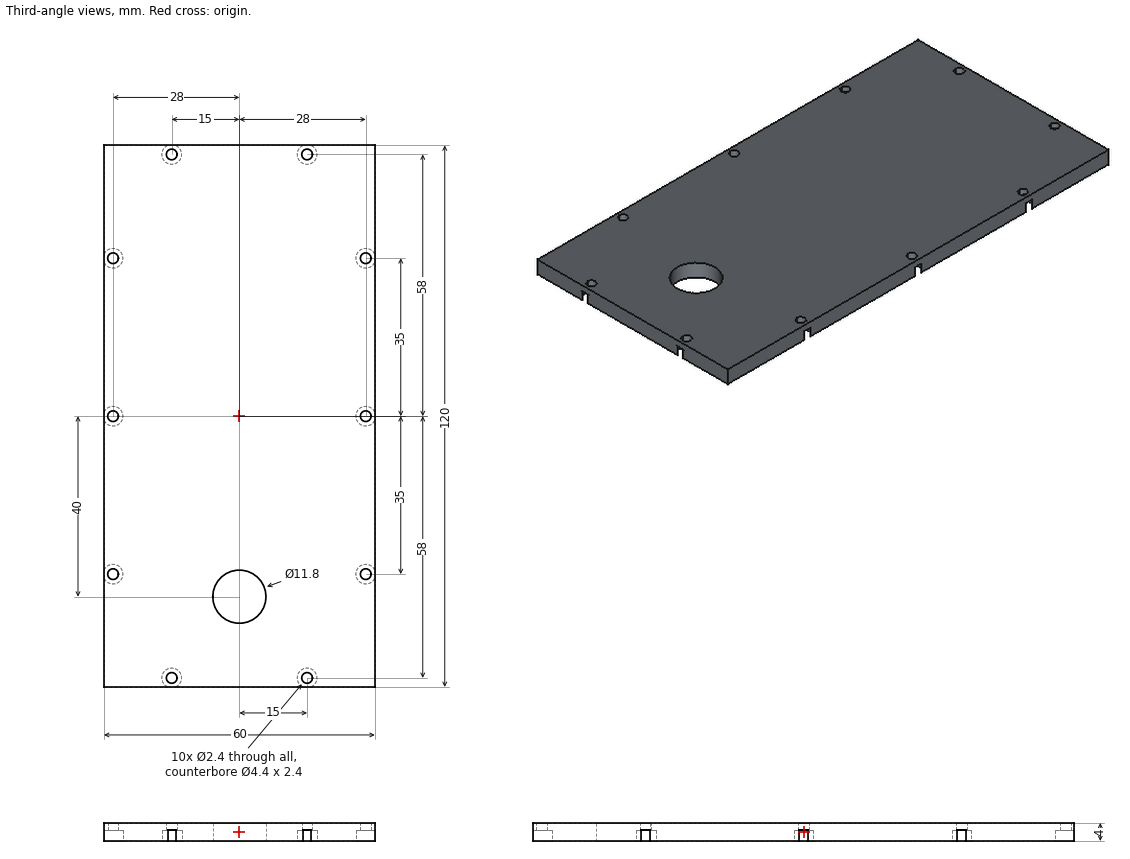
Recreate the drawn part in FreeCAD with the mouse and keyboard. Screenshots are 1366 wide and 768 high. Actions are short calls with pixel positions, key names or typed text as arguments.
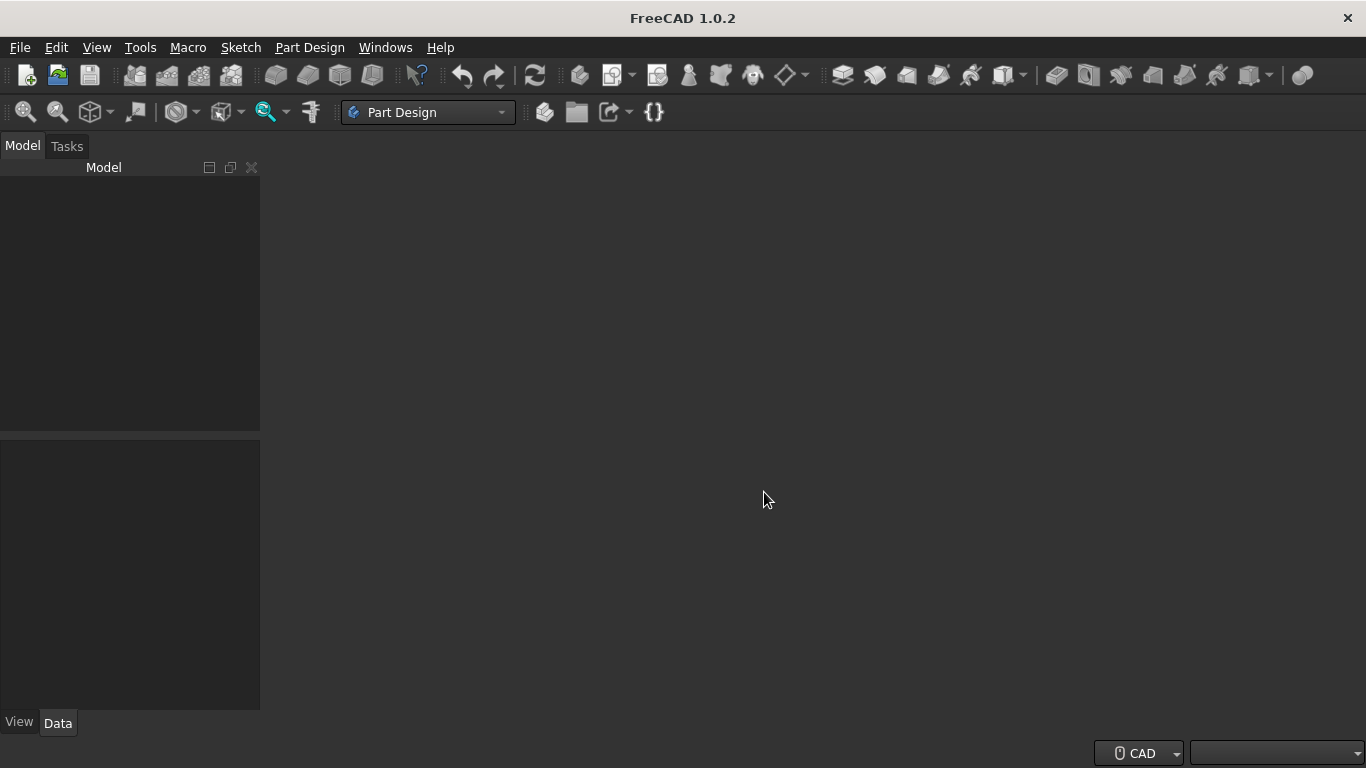
click(26, 76)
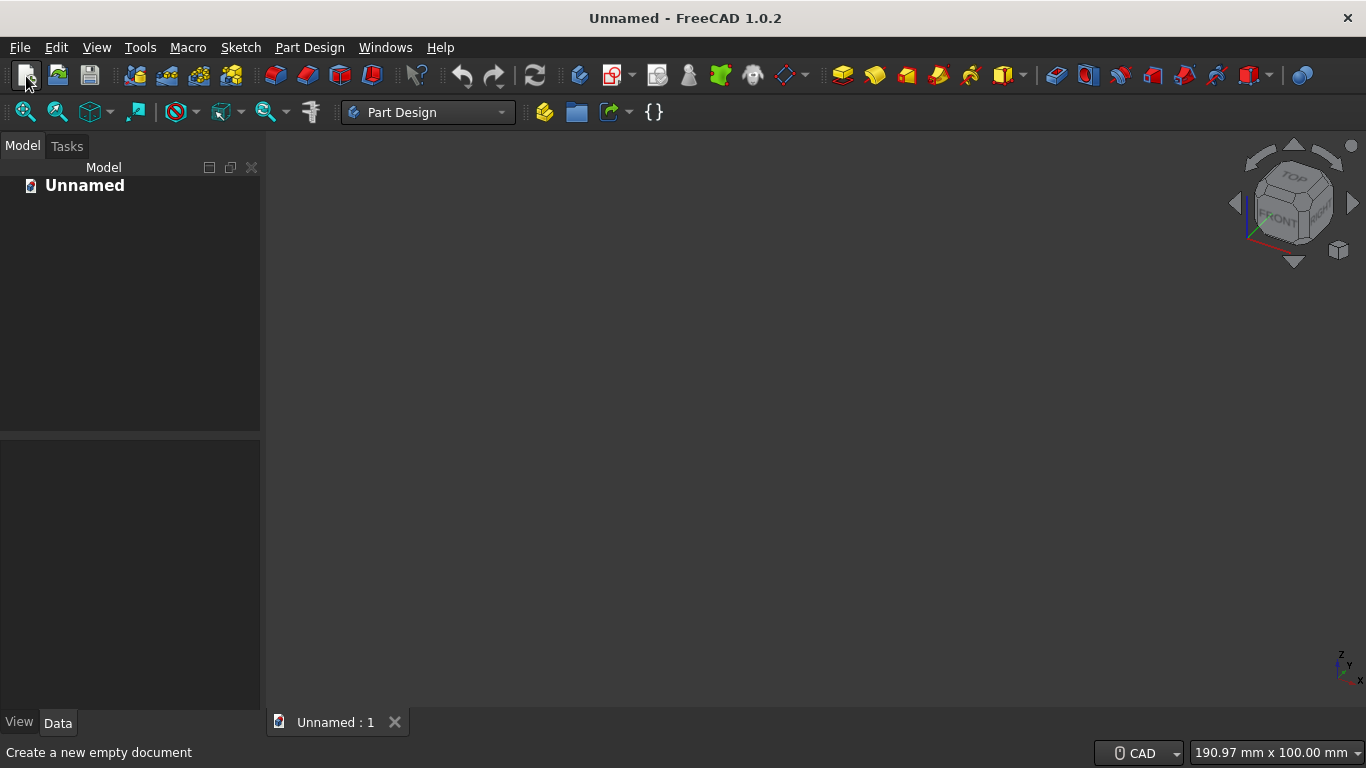
click(612, 76)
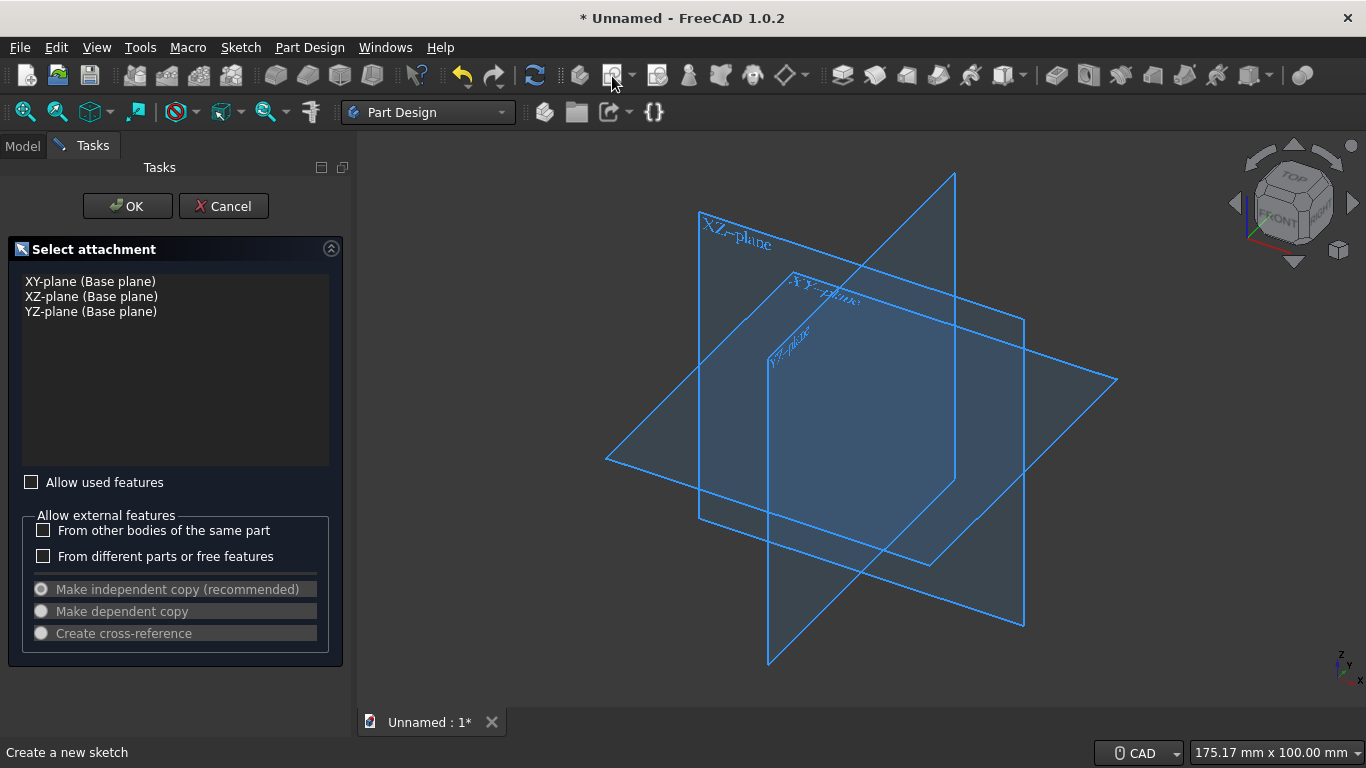
click(82, 282)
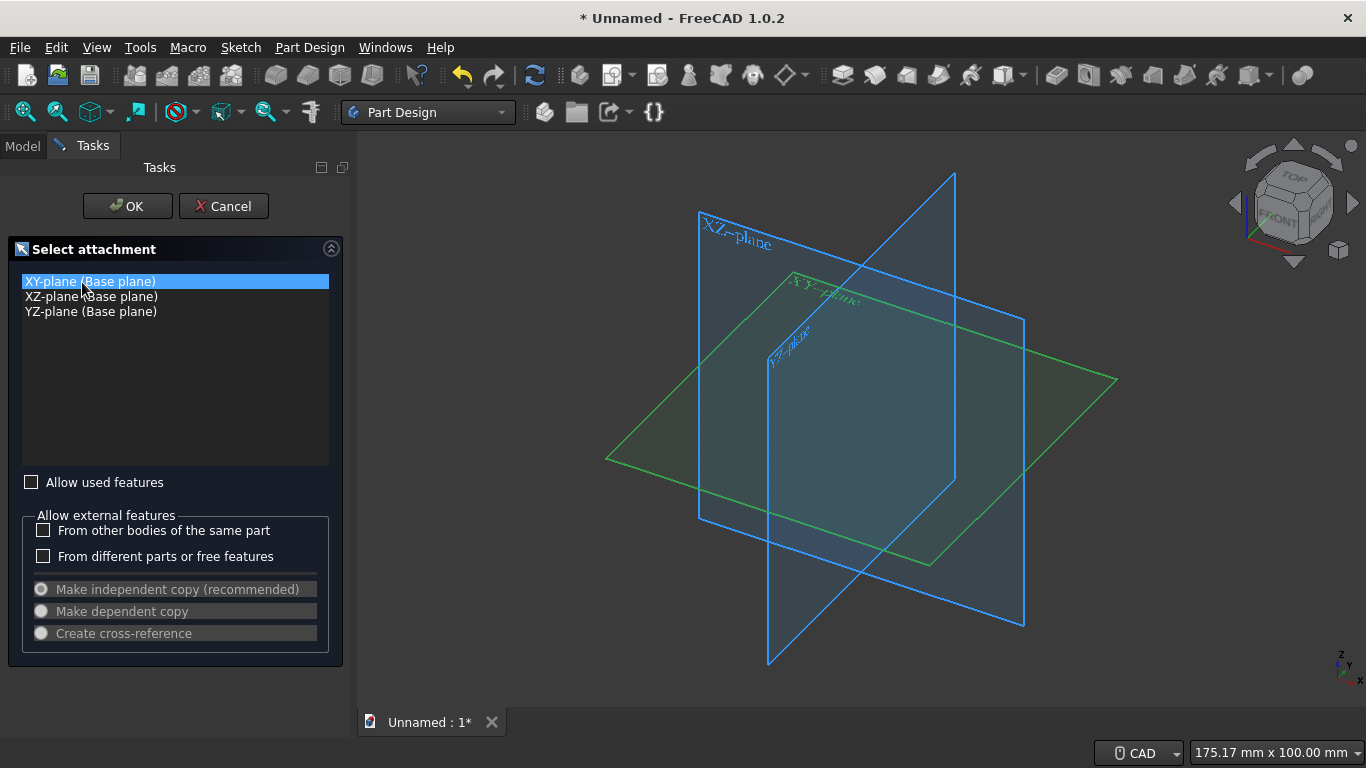
click(128, 206)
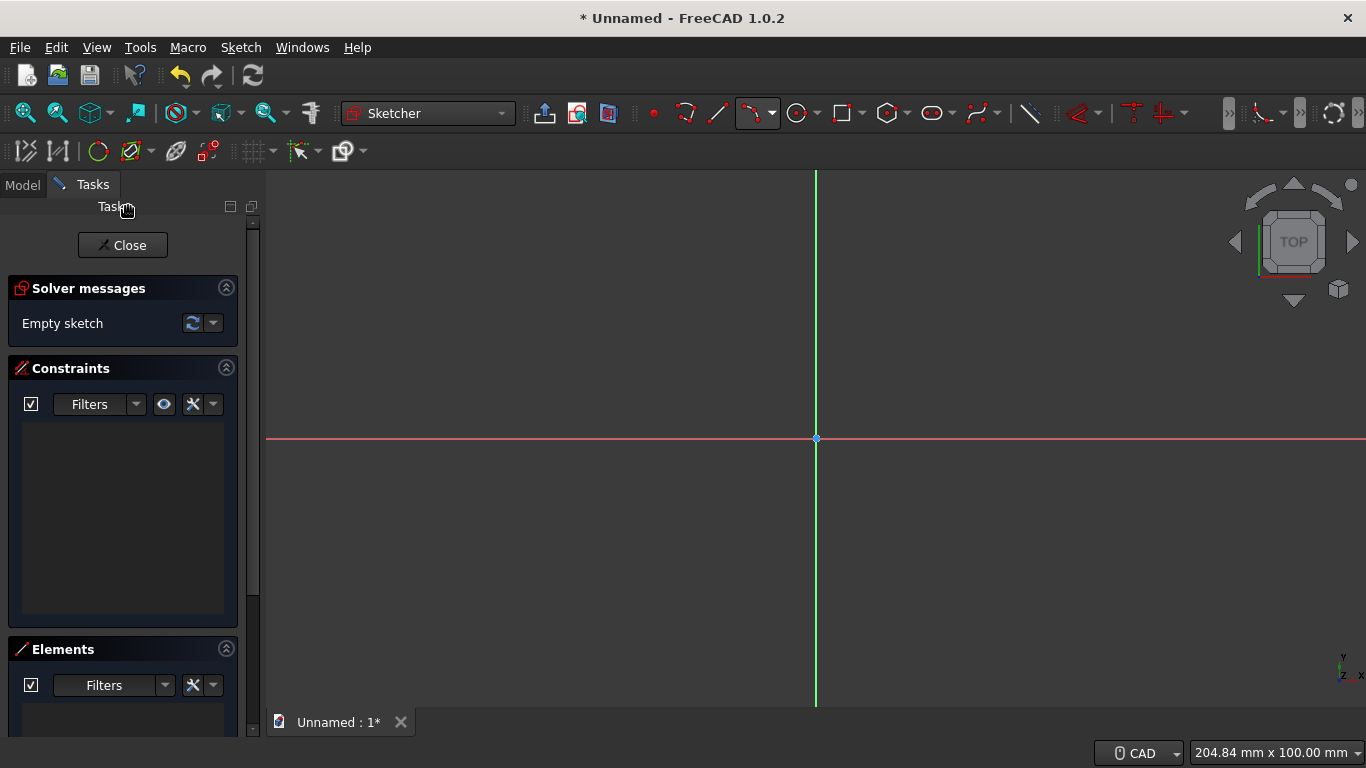
scroll(664, 438, down, 3)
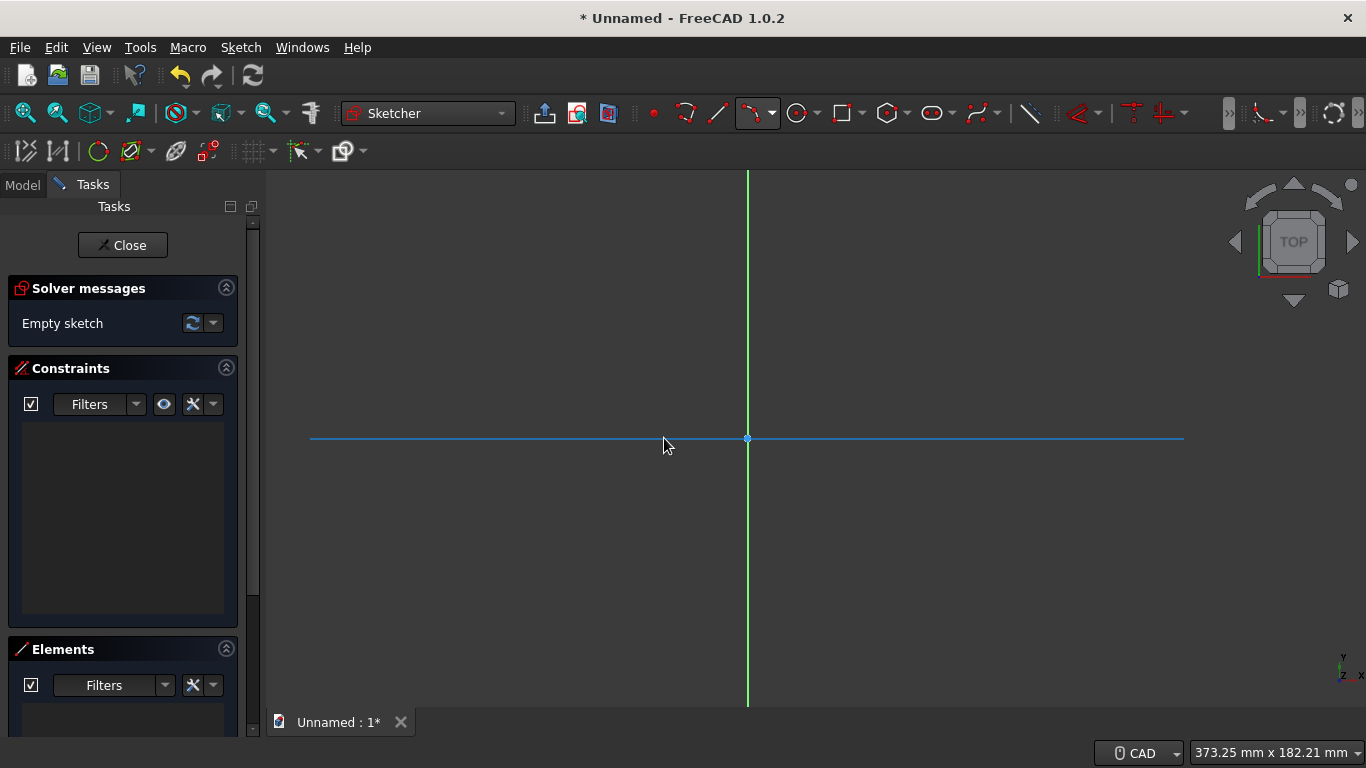
click(864, 114)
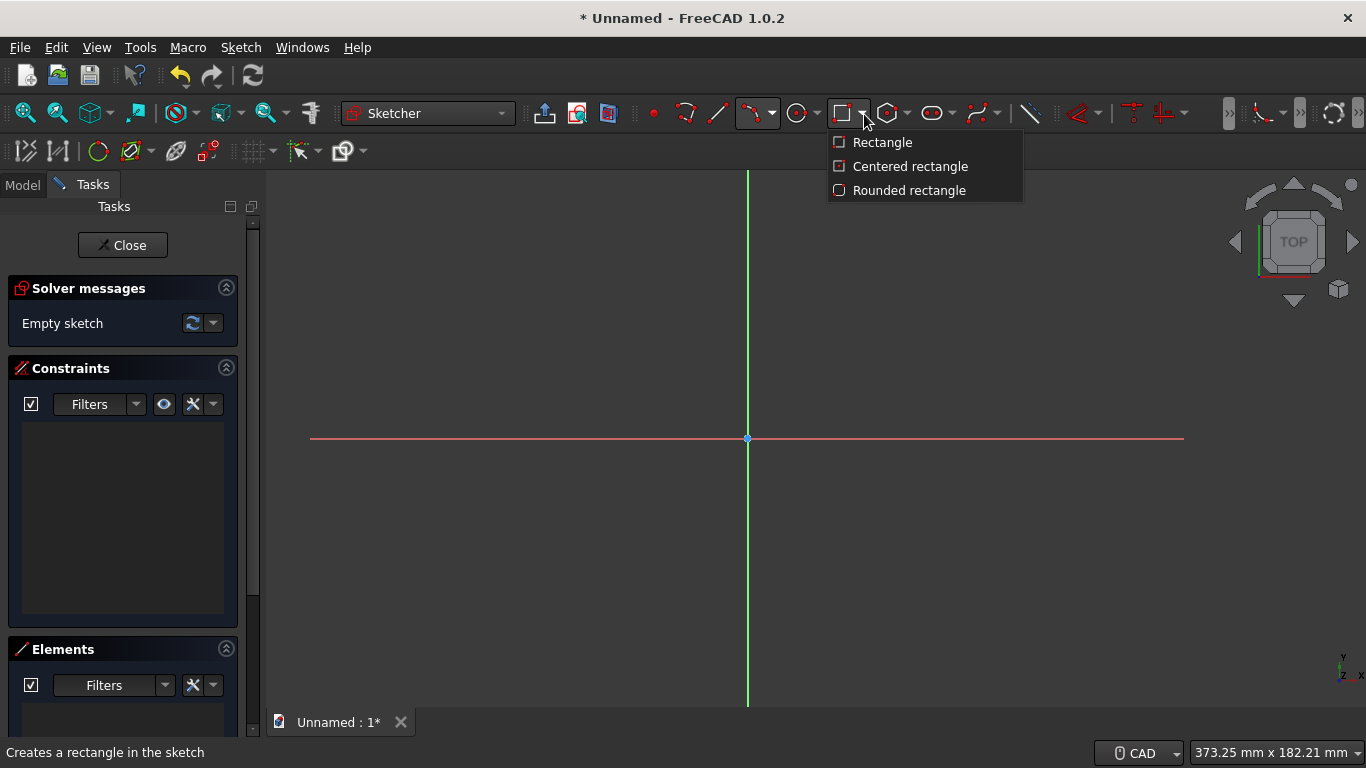
click(926, 166)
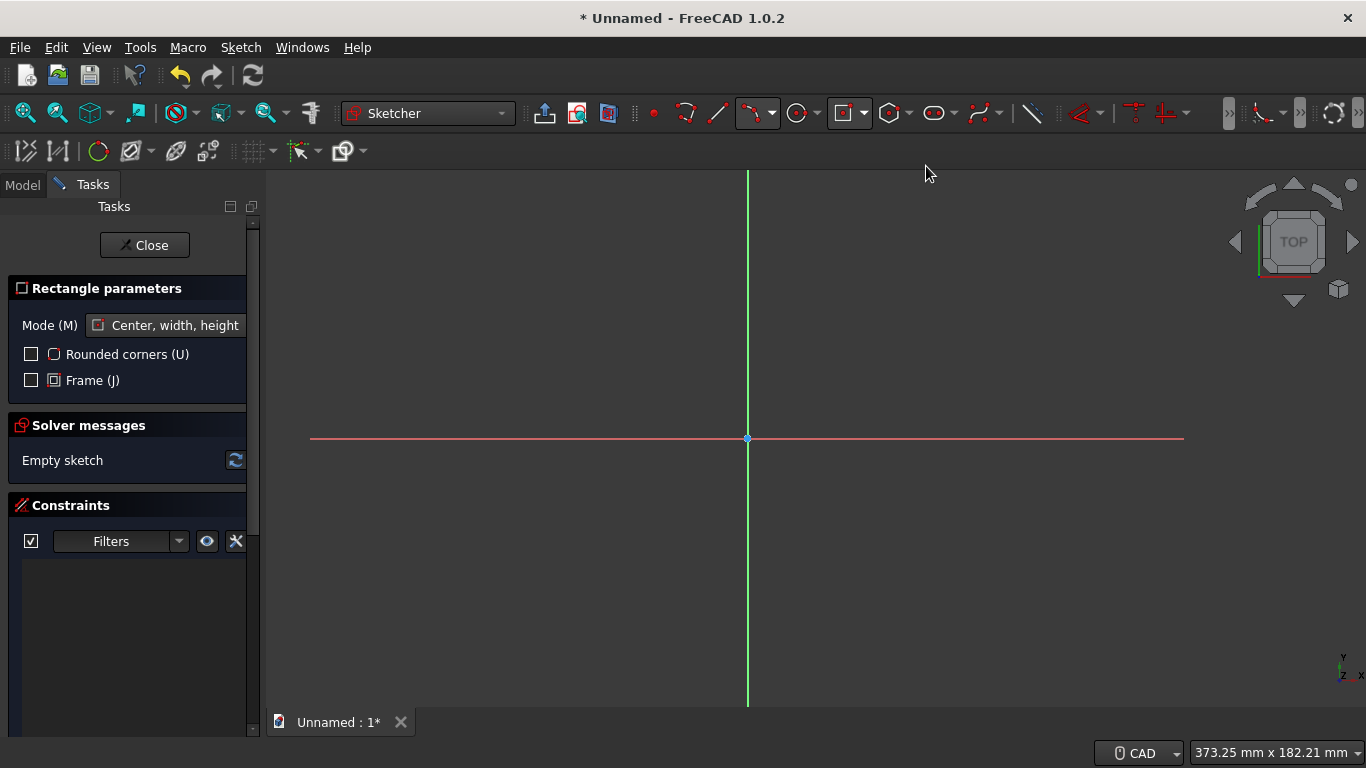
click(748, 438)
click(836, 262)
key(Escape)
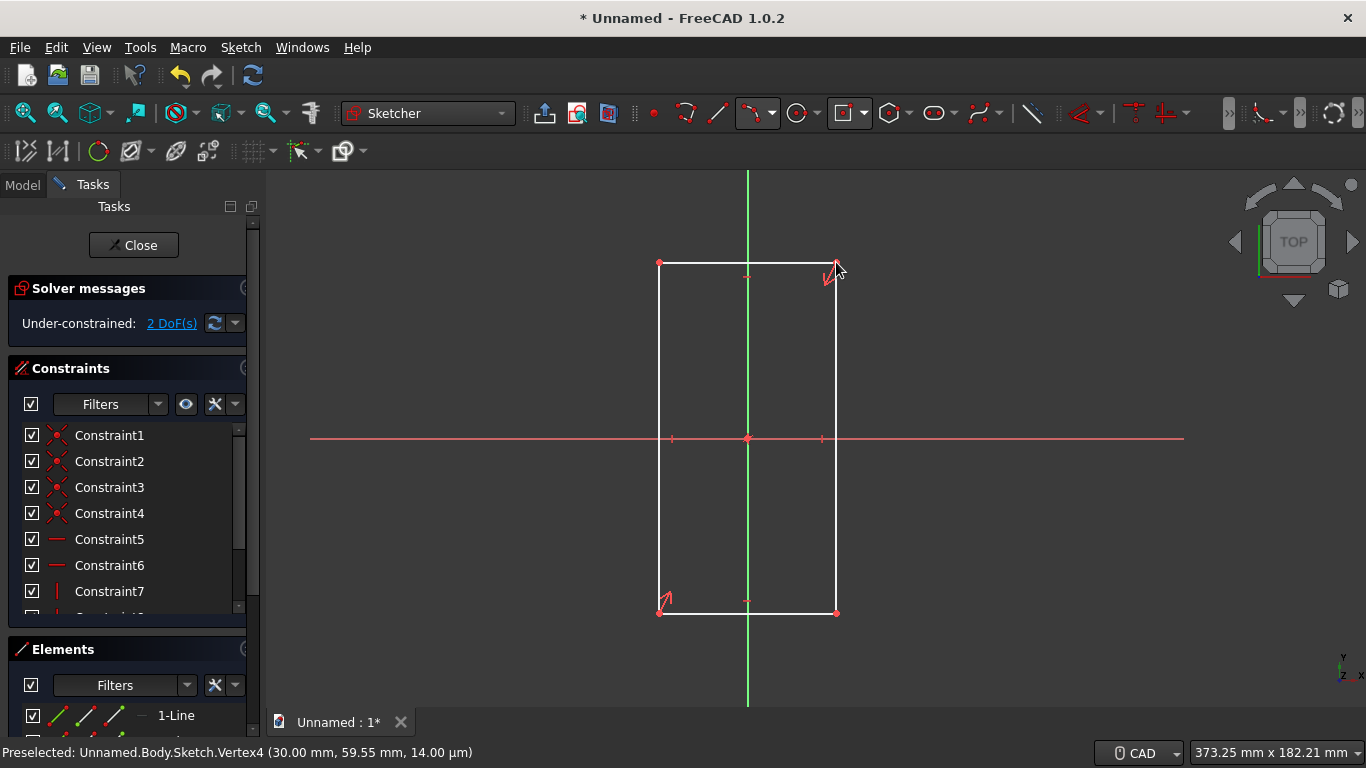
click(712, 614)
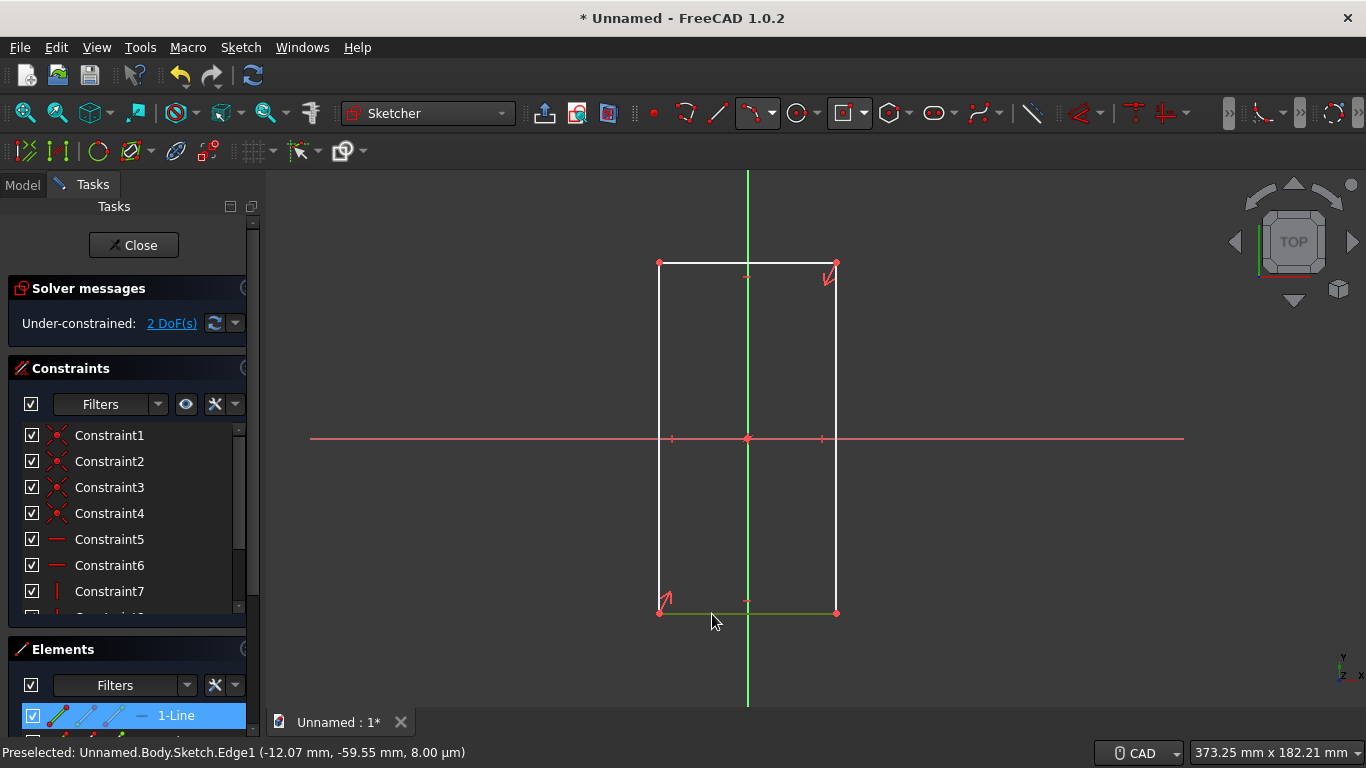
key(l)